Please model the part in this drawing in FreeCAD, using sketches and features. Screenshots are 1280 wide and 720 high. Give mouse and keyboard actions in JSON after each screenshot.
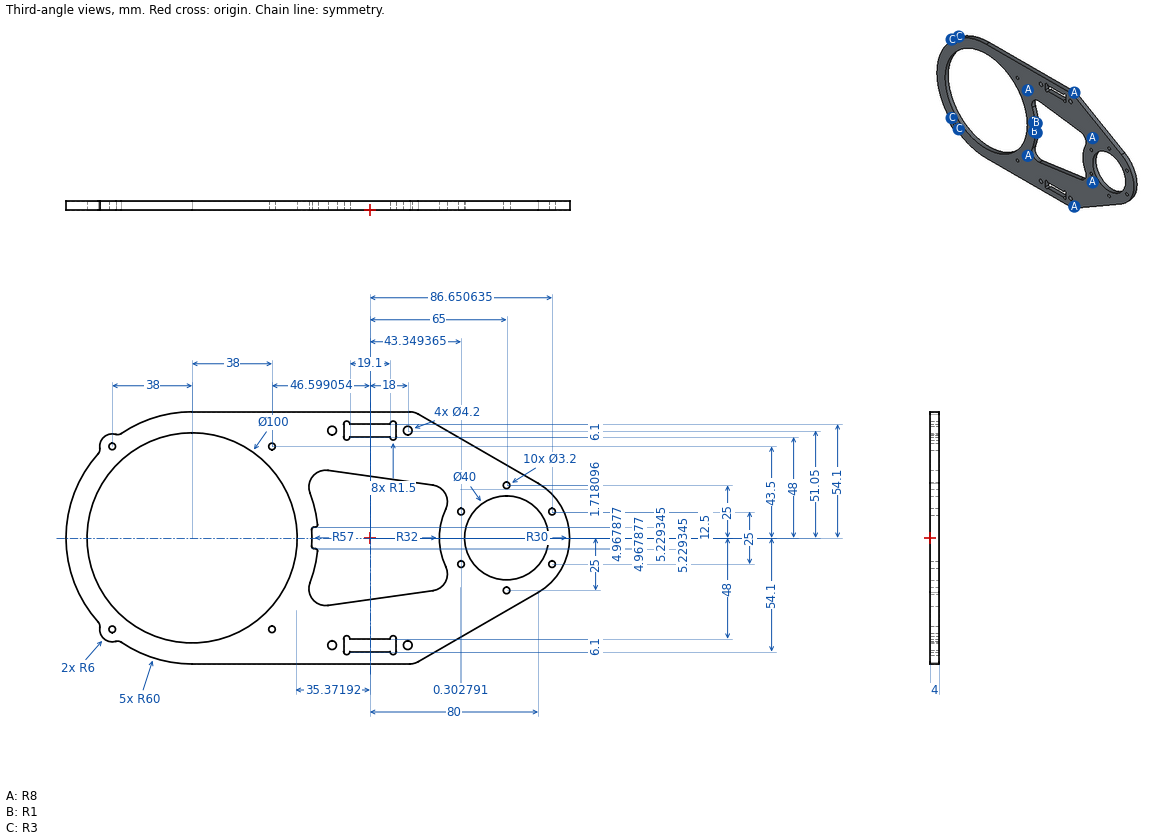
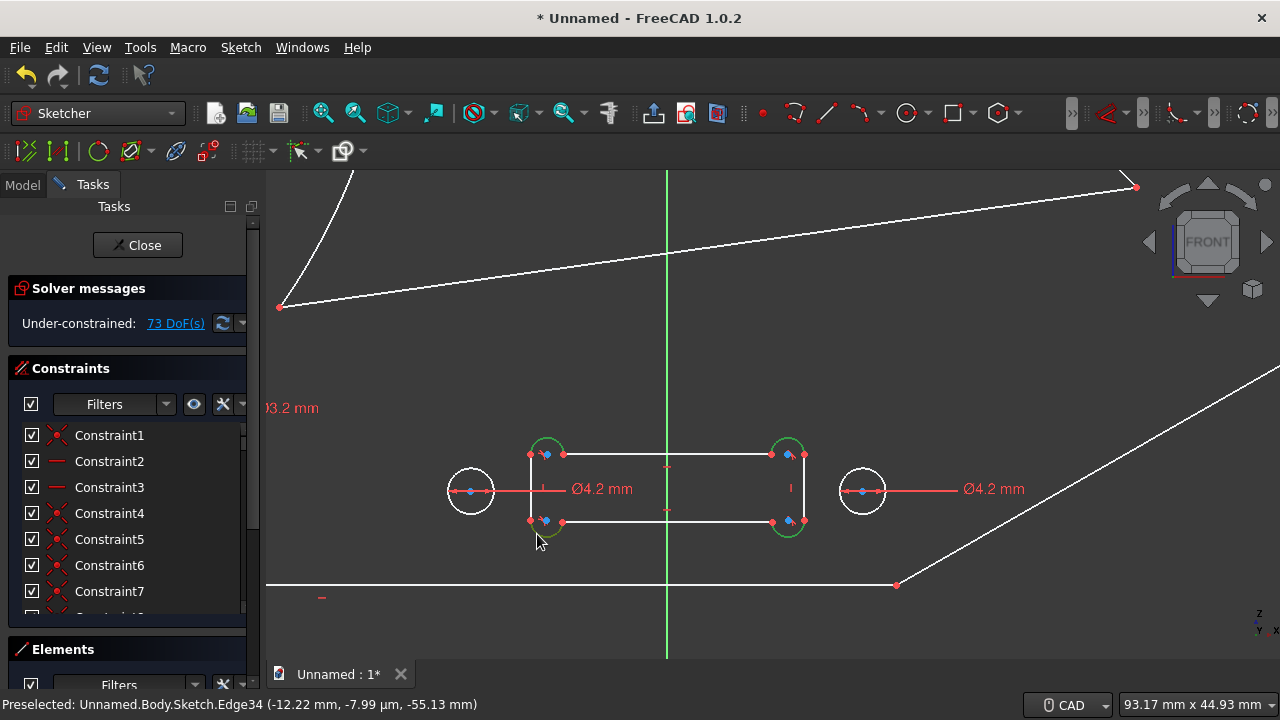
{"action": "key", "text": "e"}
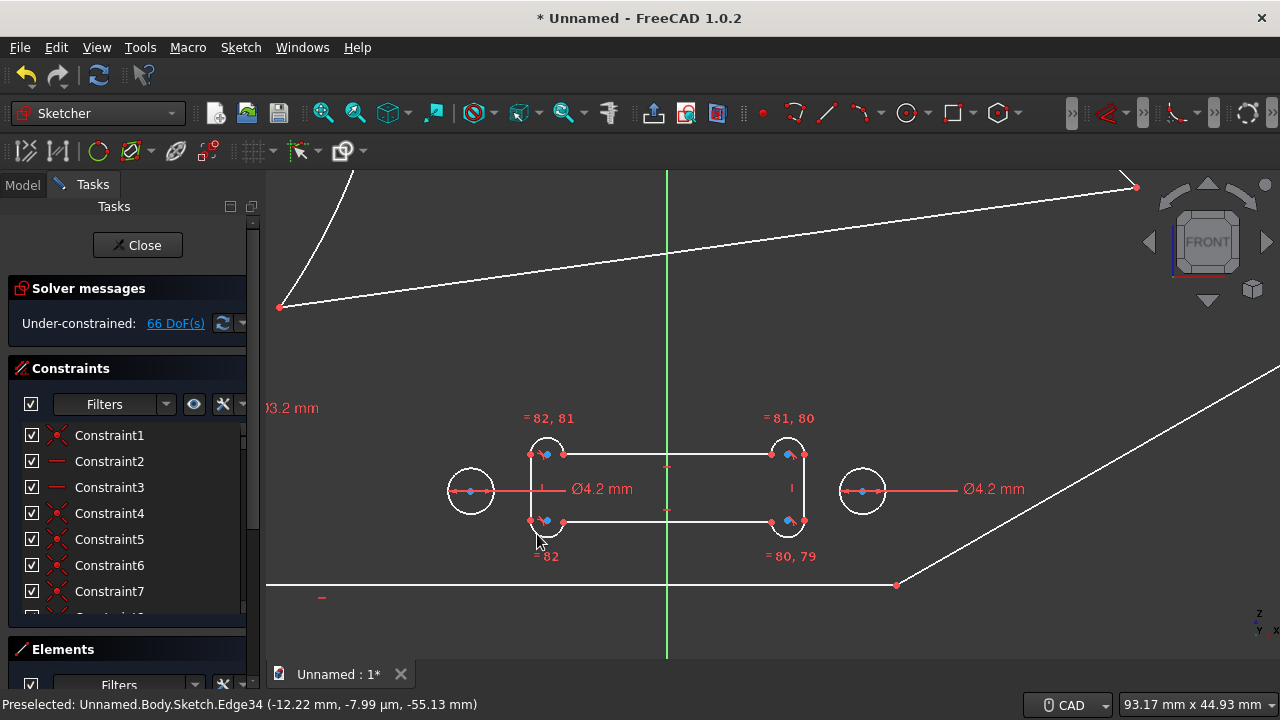
{"action": "scroll", "coordinate": [782, 537], "scroll_direction": "down", "scroll_amount": 8}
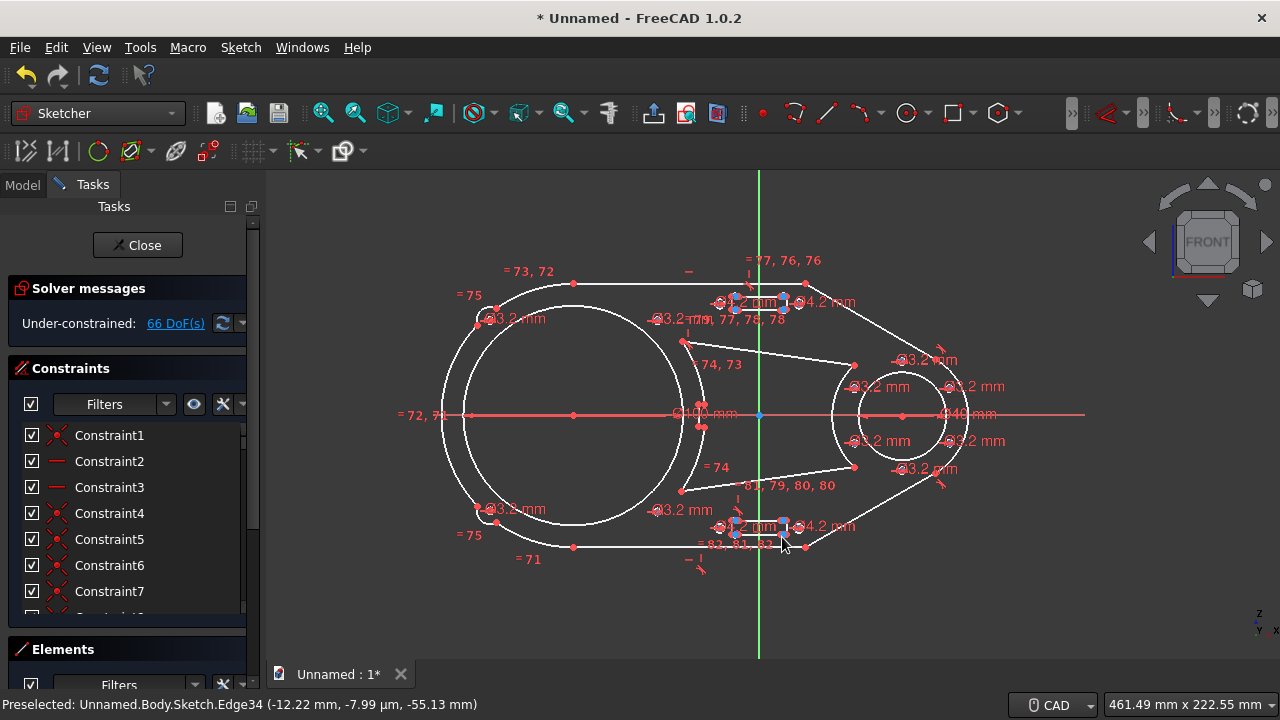
{"action": "left_click", "coordinate": [573, 416]}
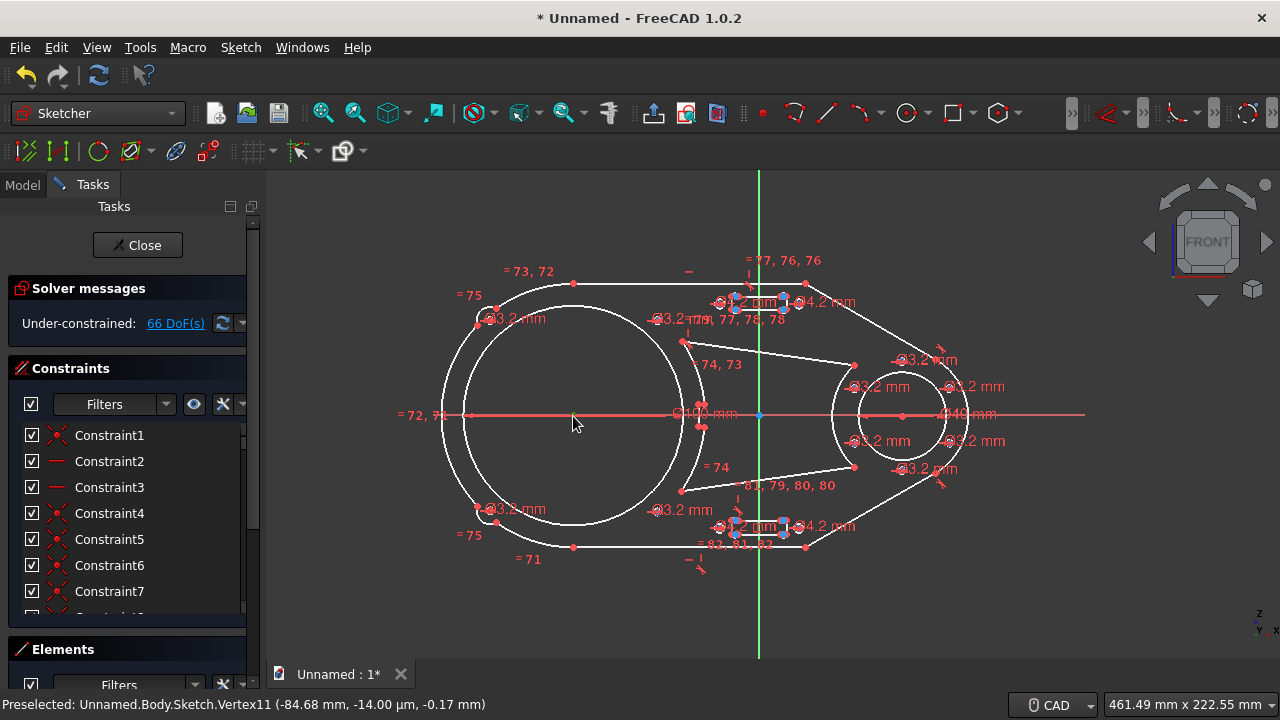
{"action": "left_click", "coordinate": [529, 415]}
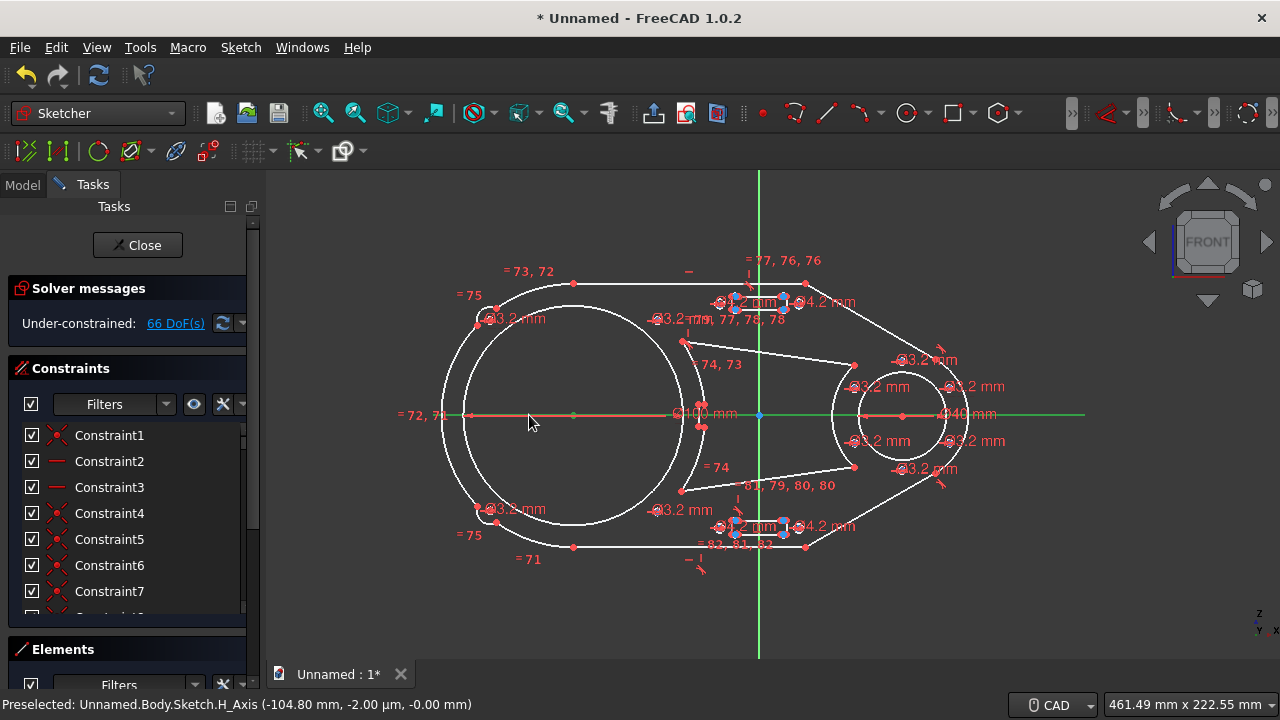
{"action": "key", "text": "c"}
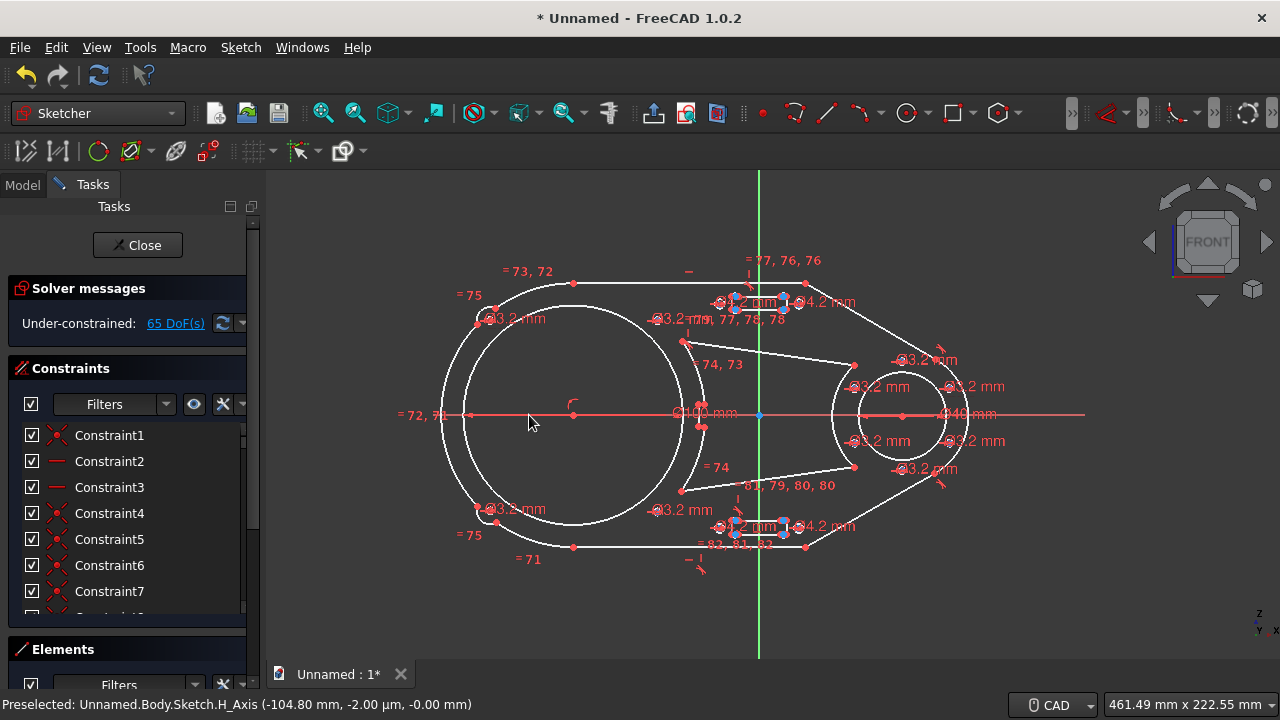
{"action": "left_click", "coordinate": [902, 416]}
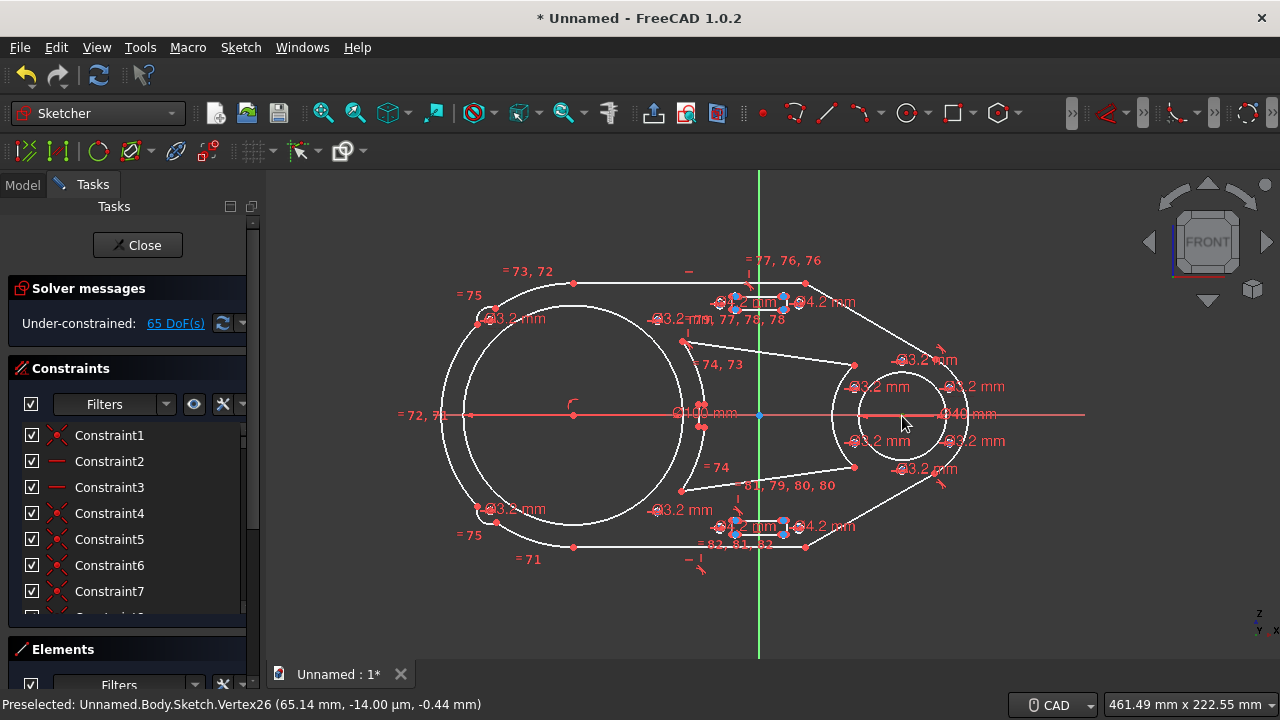
{"action": "left_click", "coordinate": [529, 415]}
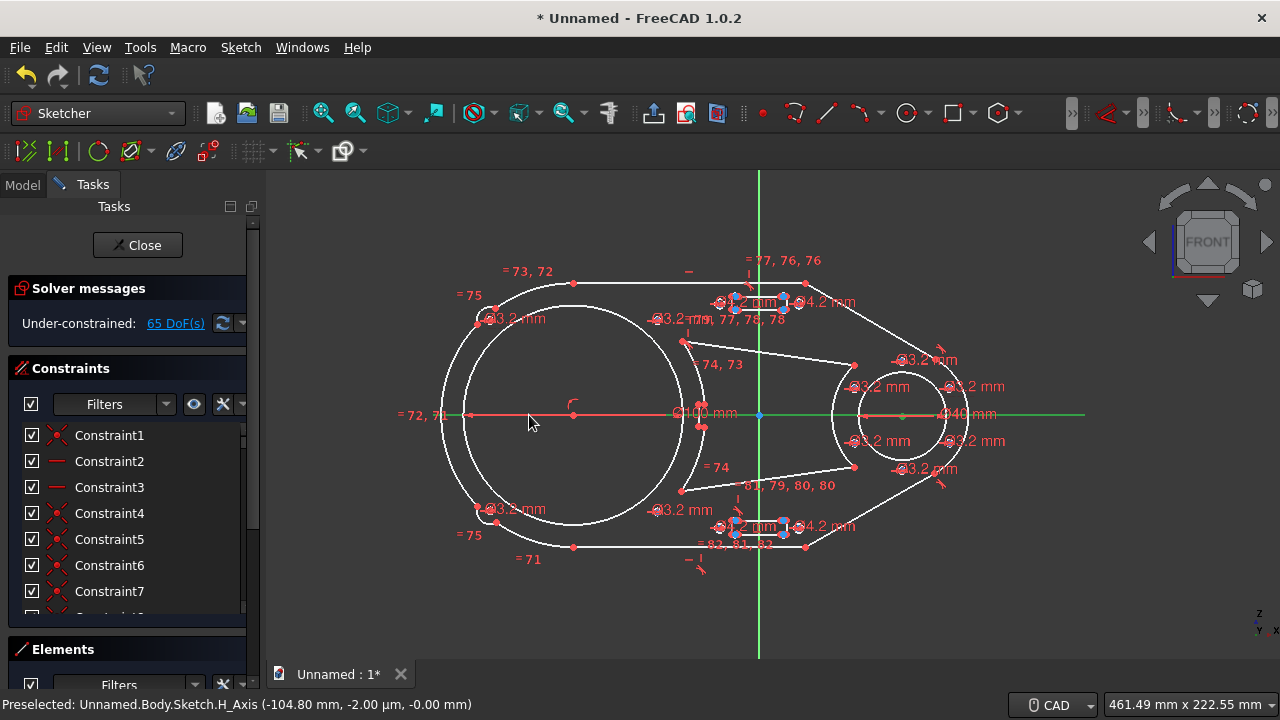
{"action": "key", "text": "c"}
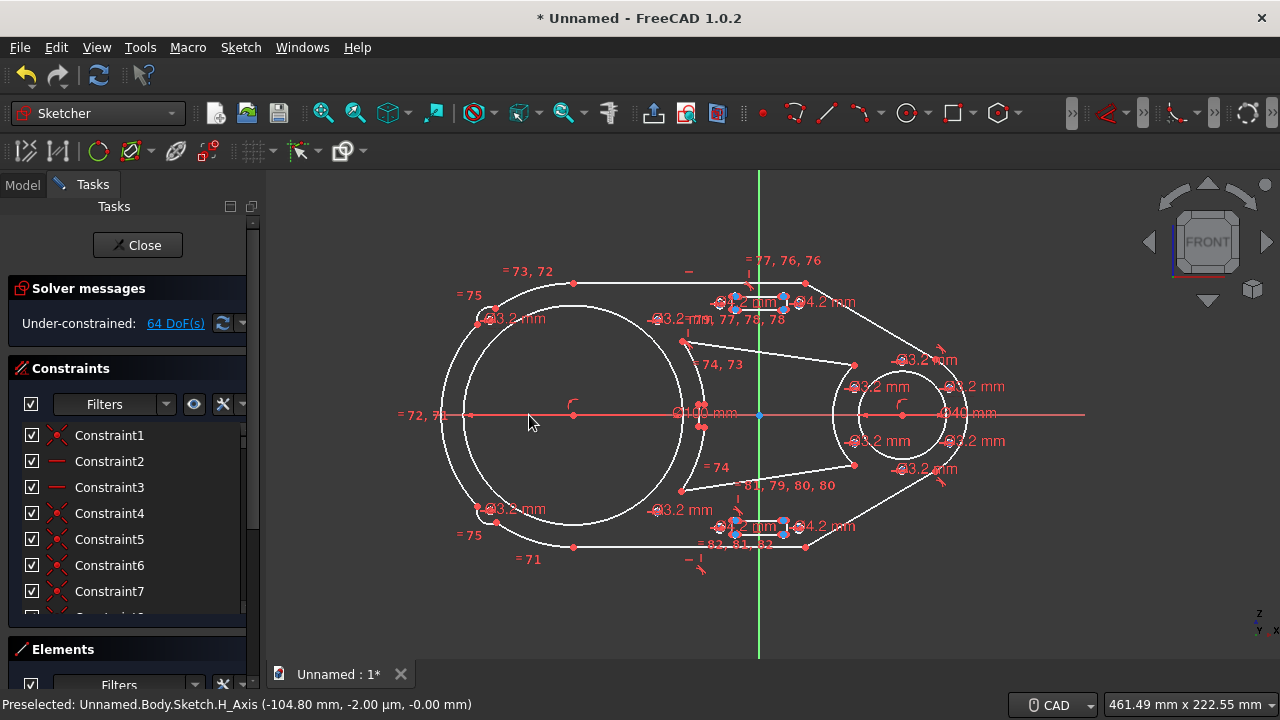
{"action": "left_click", "coordinate": [902, 362]}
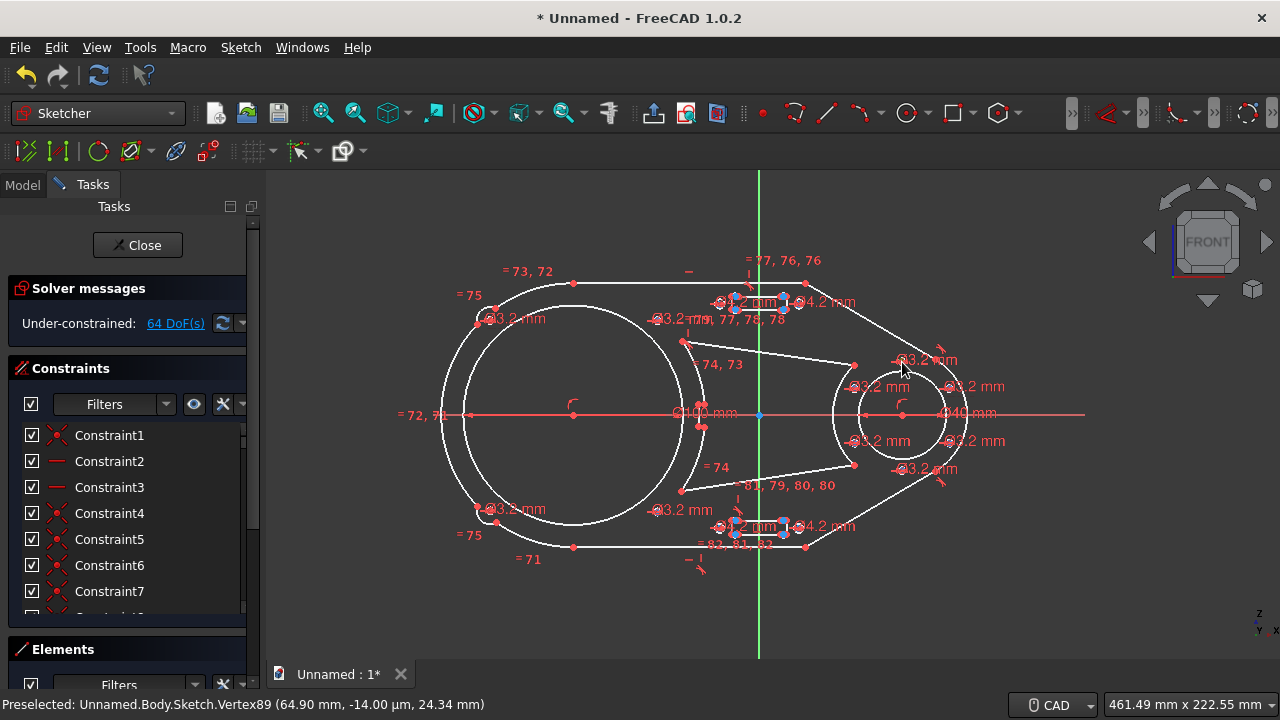
{"action": "left_click", "coordinate": [902, 415]}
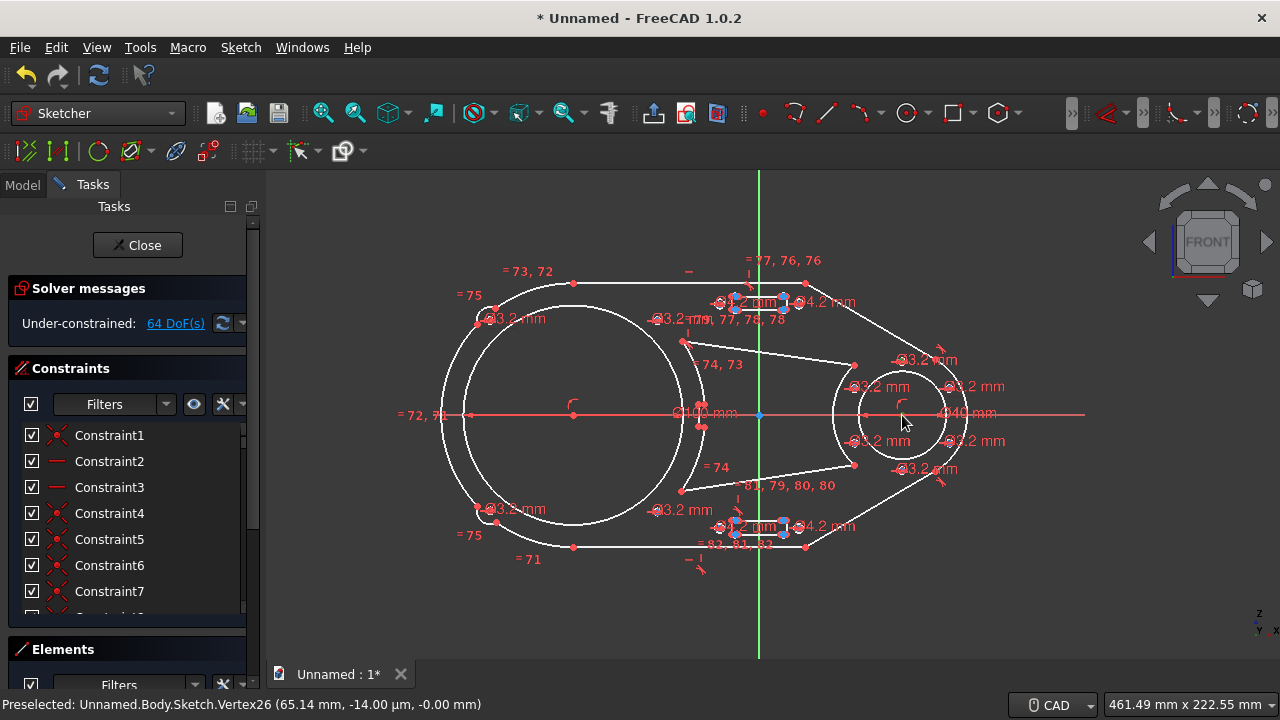
{"action": "key", "text": "v"}